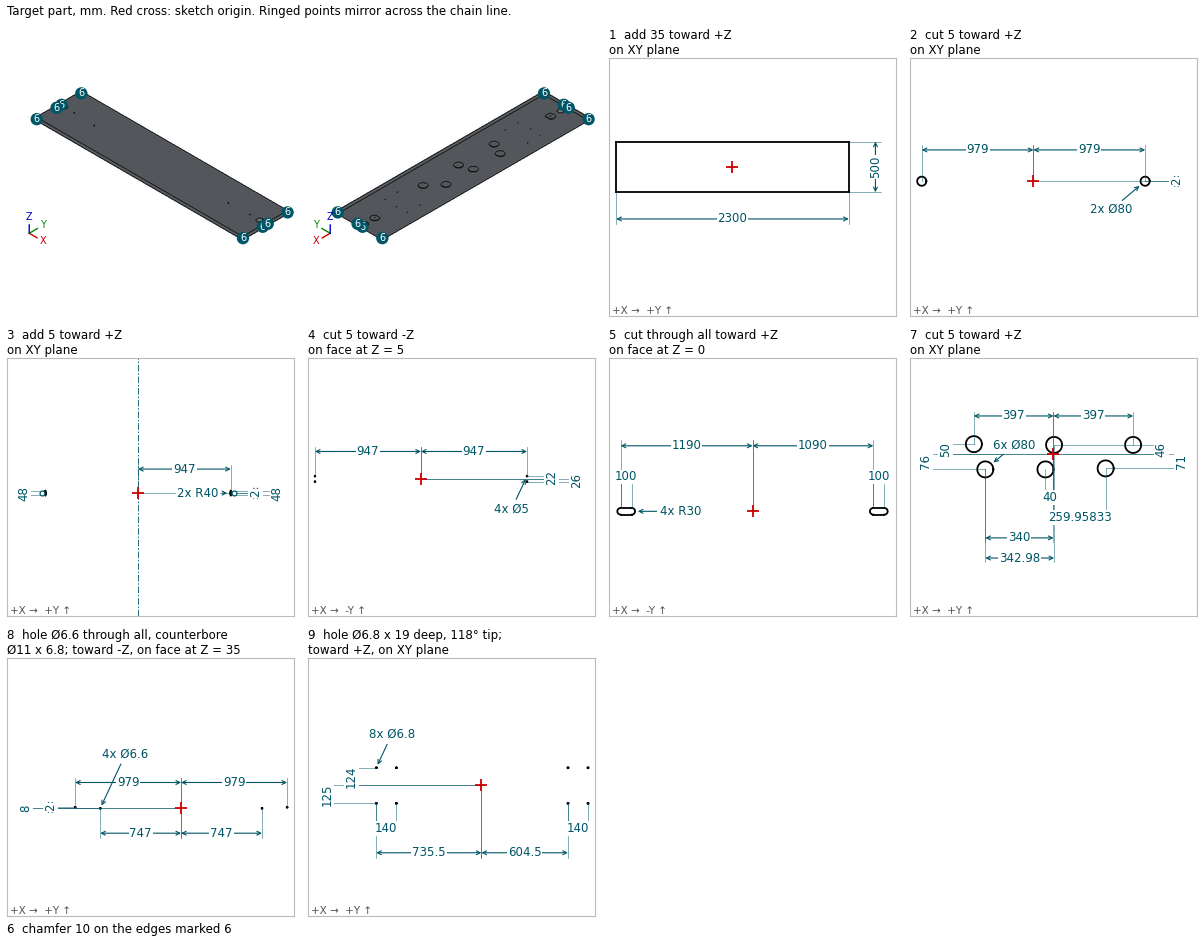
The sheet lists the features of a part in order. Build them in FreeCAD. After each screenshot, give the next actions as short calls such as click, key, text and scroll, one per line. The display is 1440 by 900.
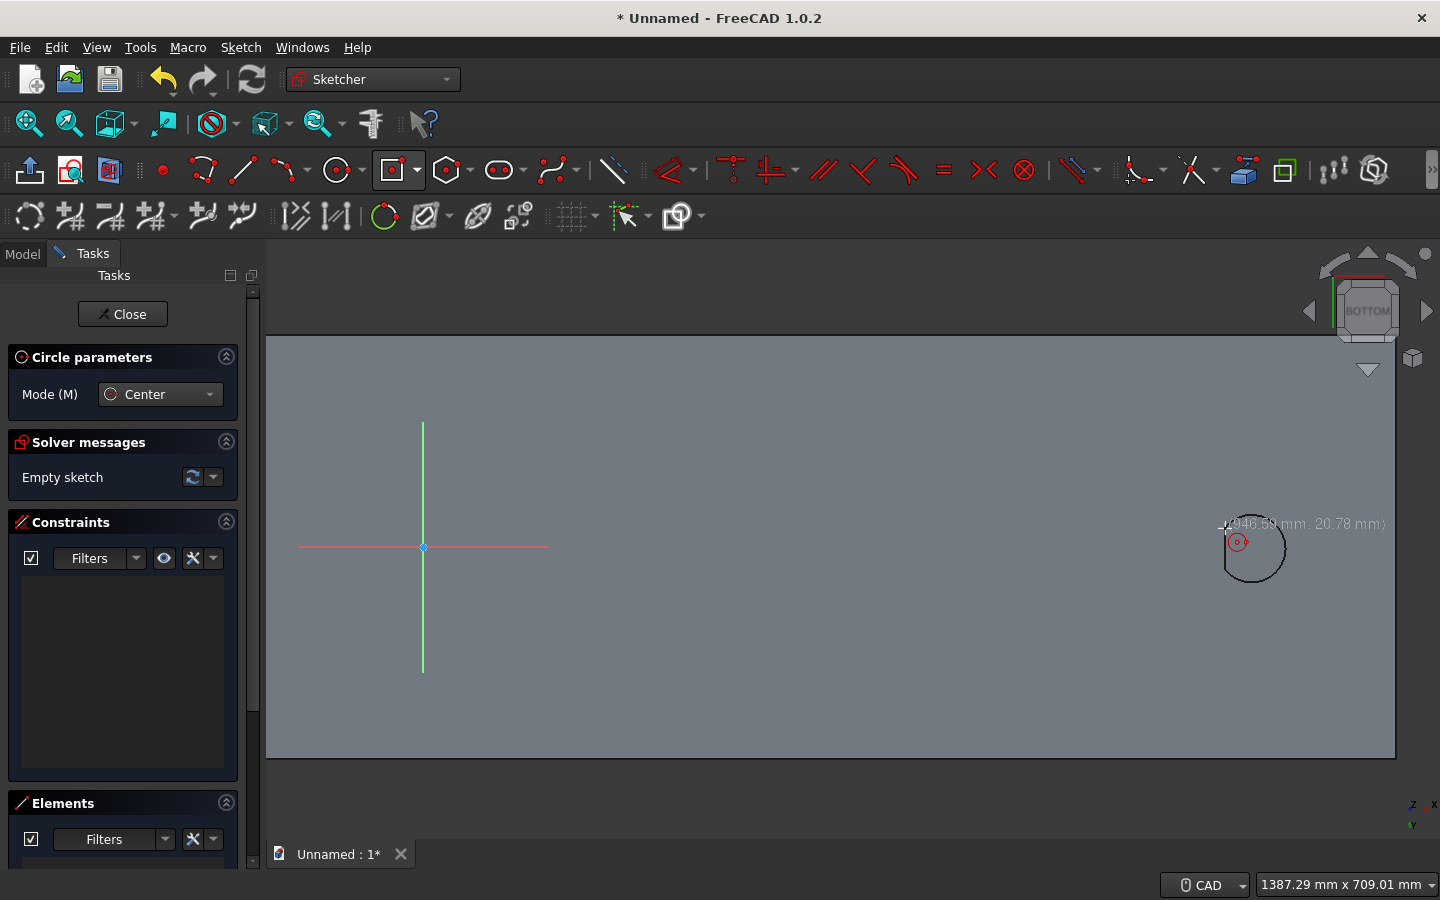
click(1225, 528)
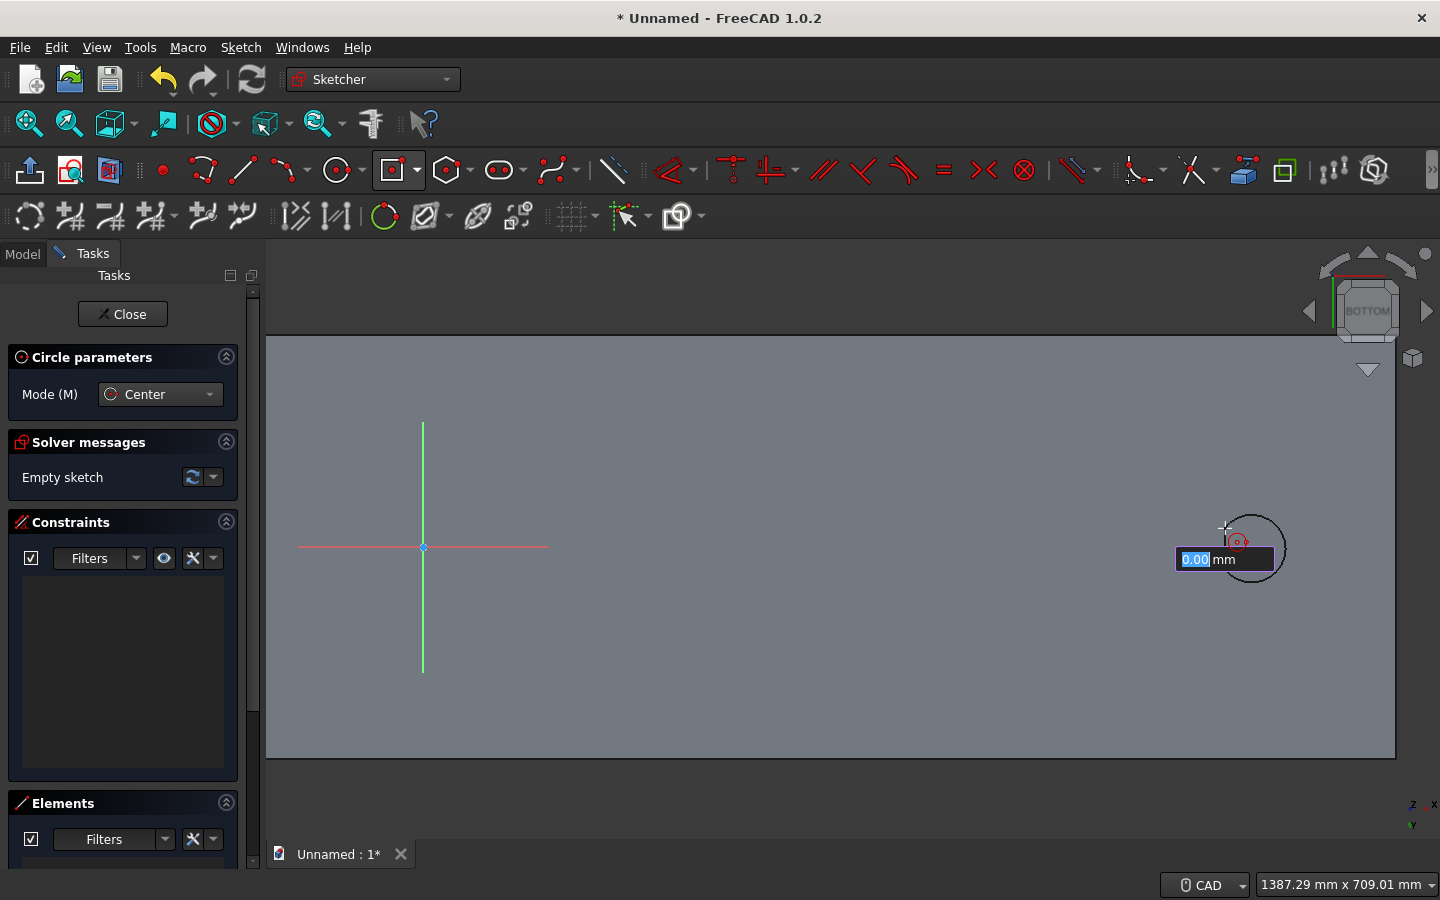
scroll(1226, 527, up, 11)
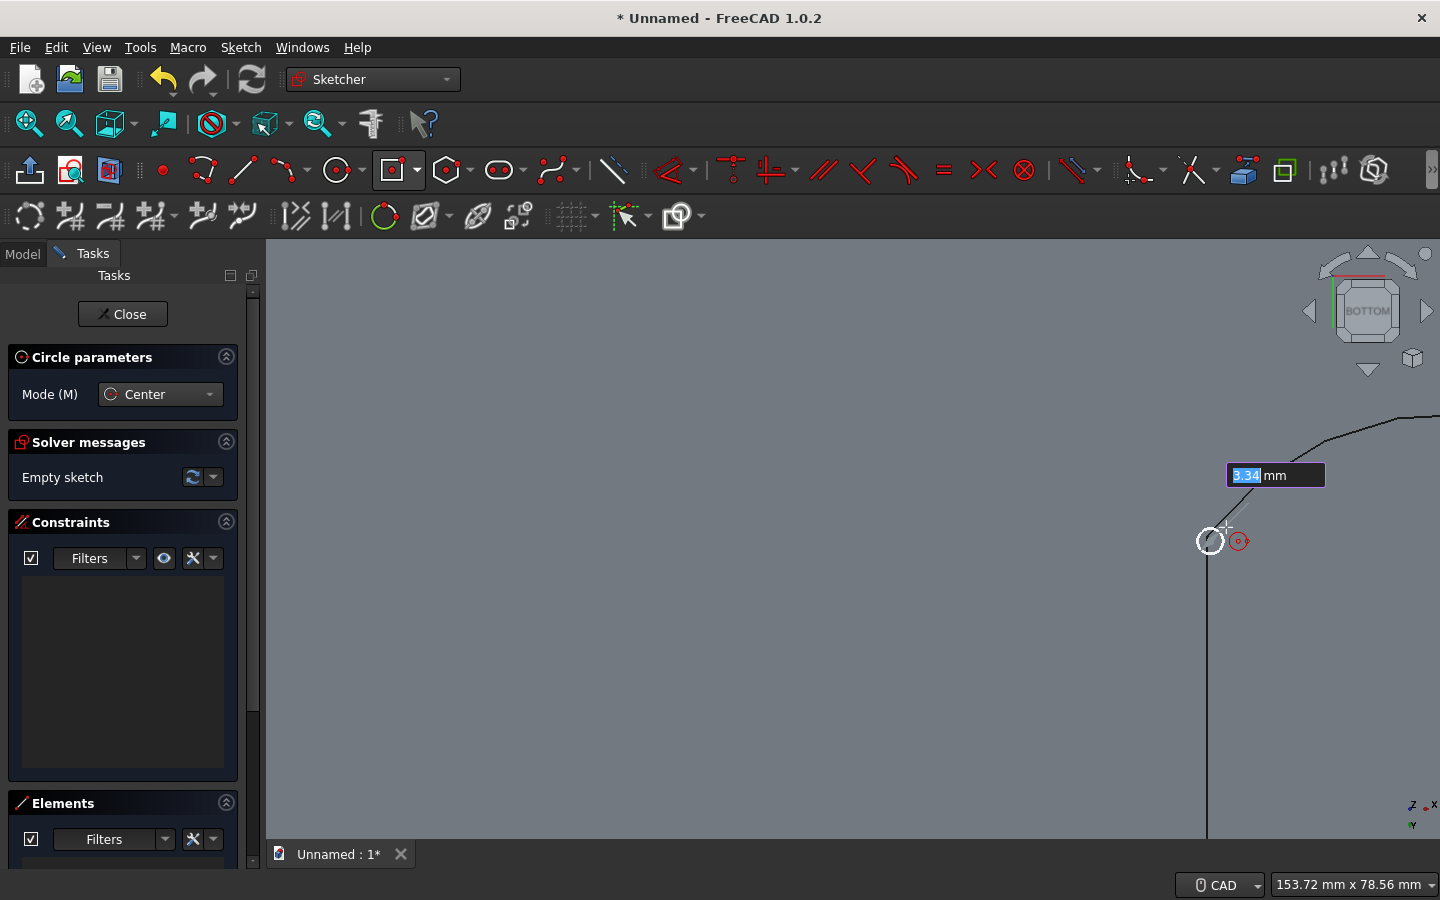
click(1221, 522)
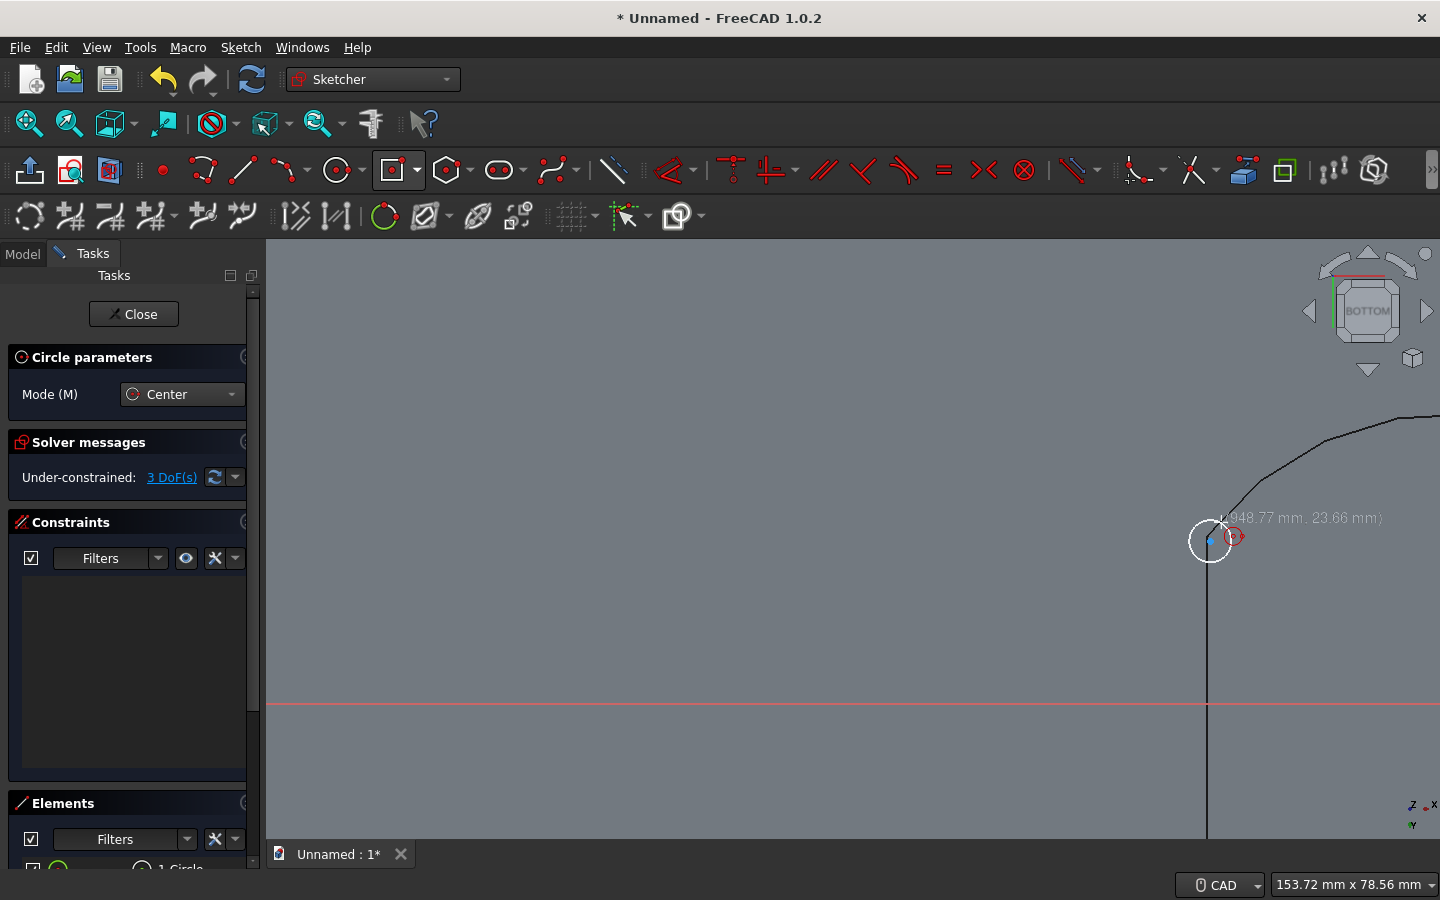
scroll(1141, 530, down, 15)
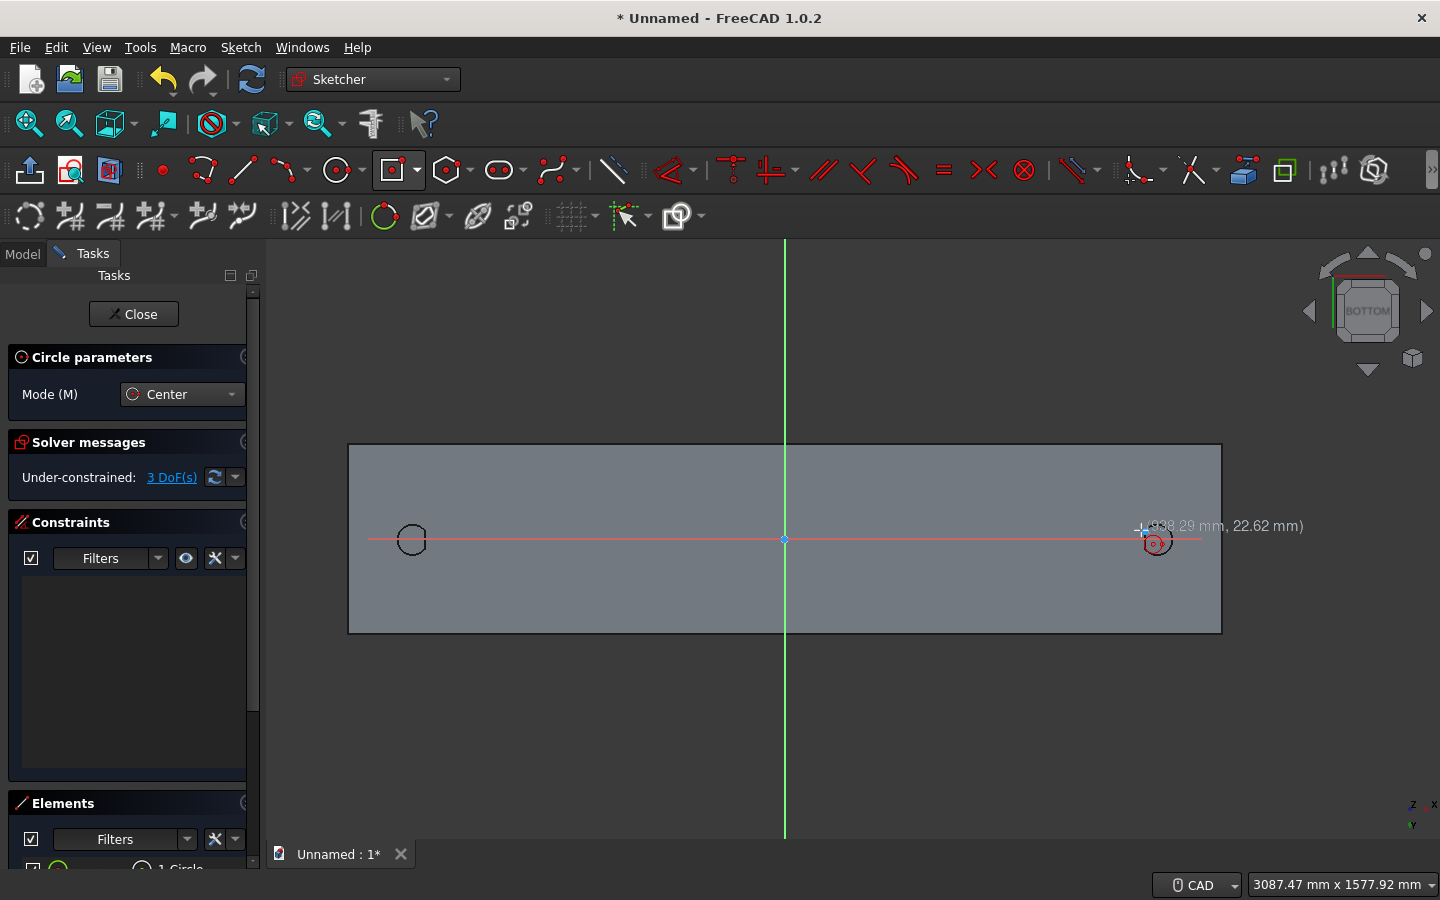
scroll(1145, 549, up, 16)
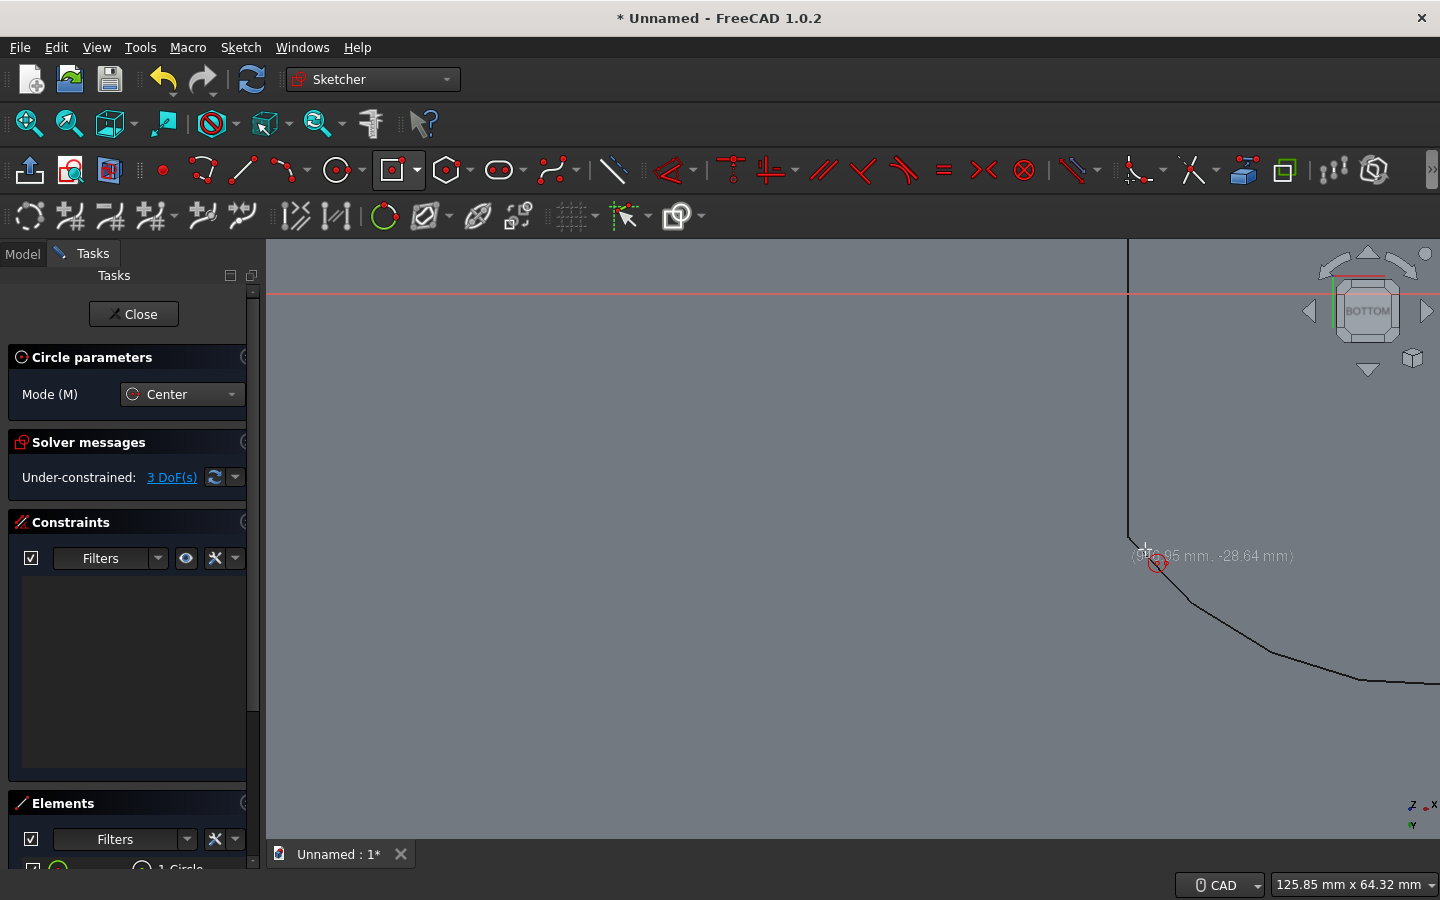
scroll(1229, 551, down, 15)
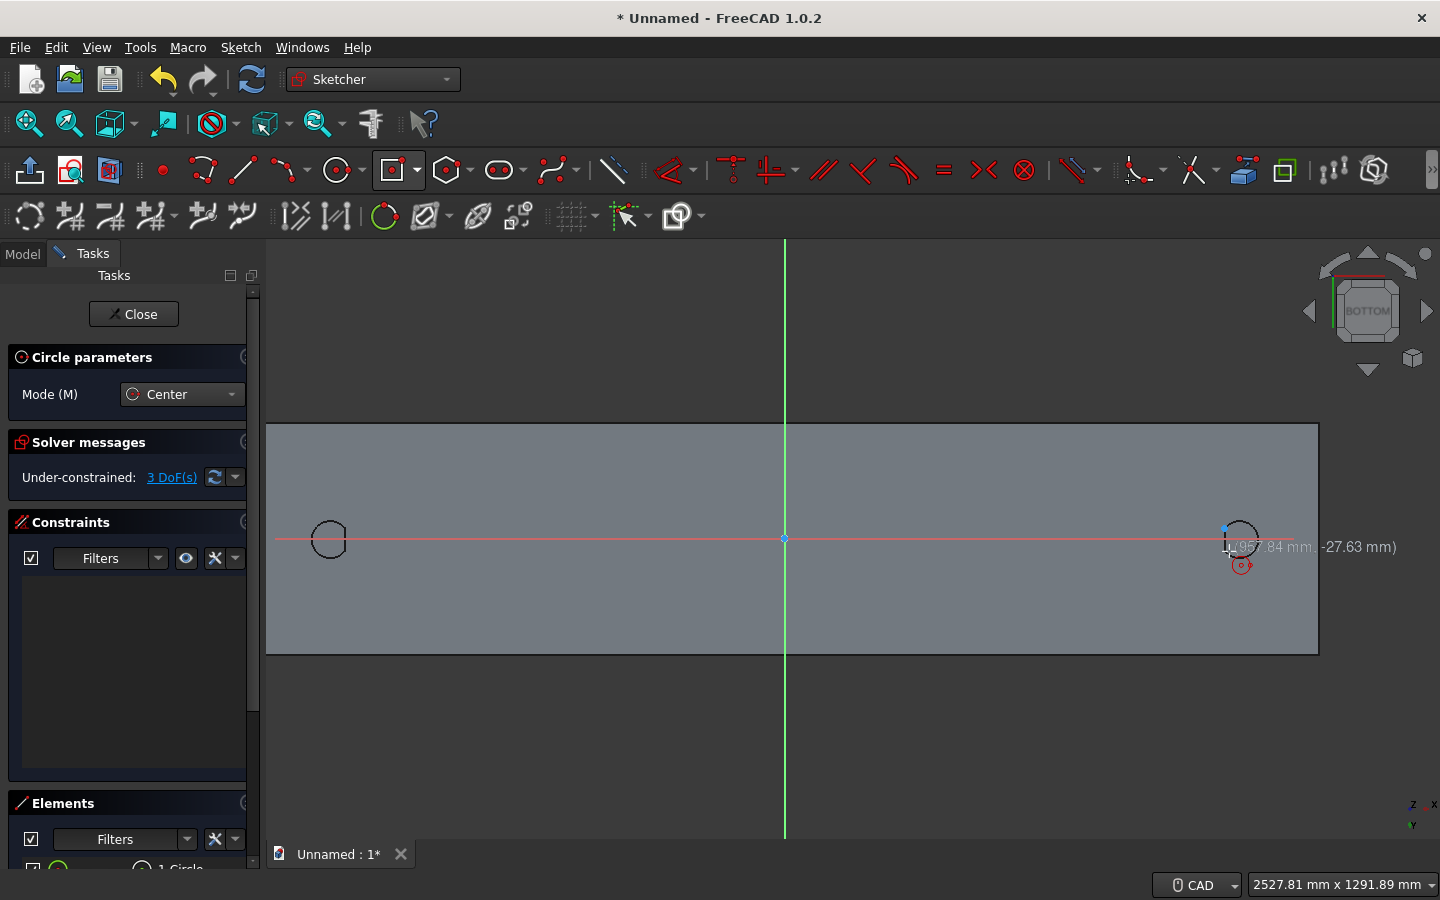
scroll(1225, 551, up, 2)